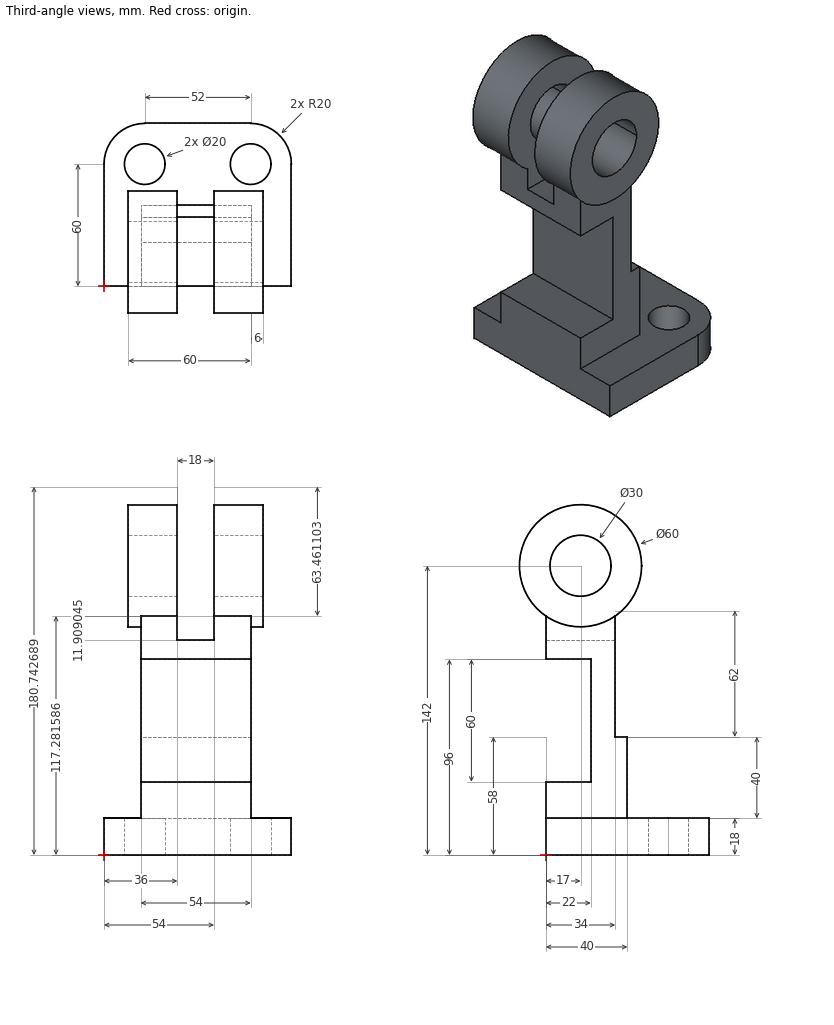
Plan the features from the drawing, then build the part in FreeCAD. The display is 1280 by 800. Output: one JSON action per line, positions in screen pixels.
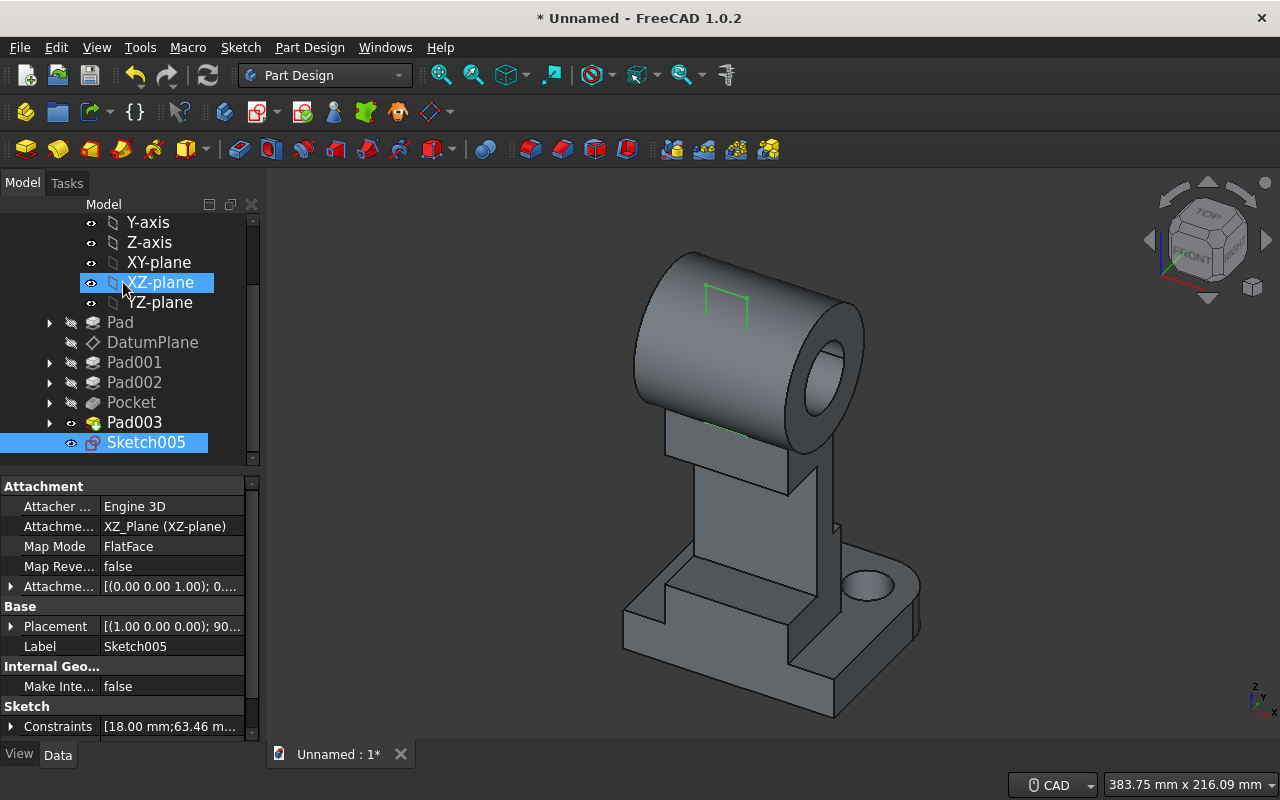
{"action": "left_click", "coordinate": [240, 150]}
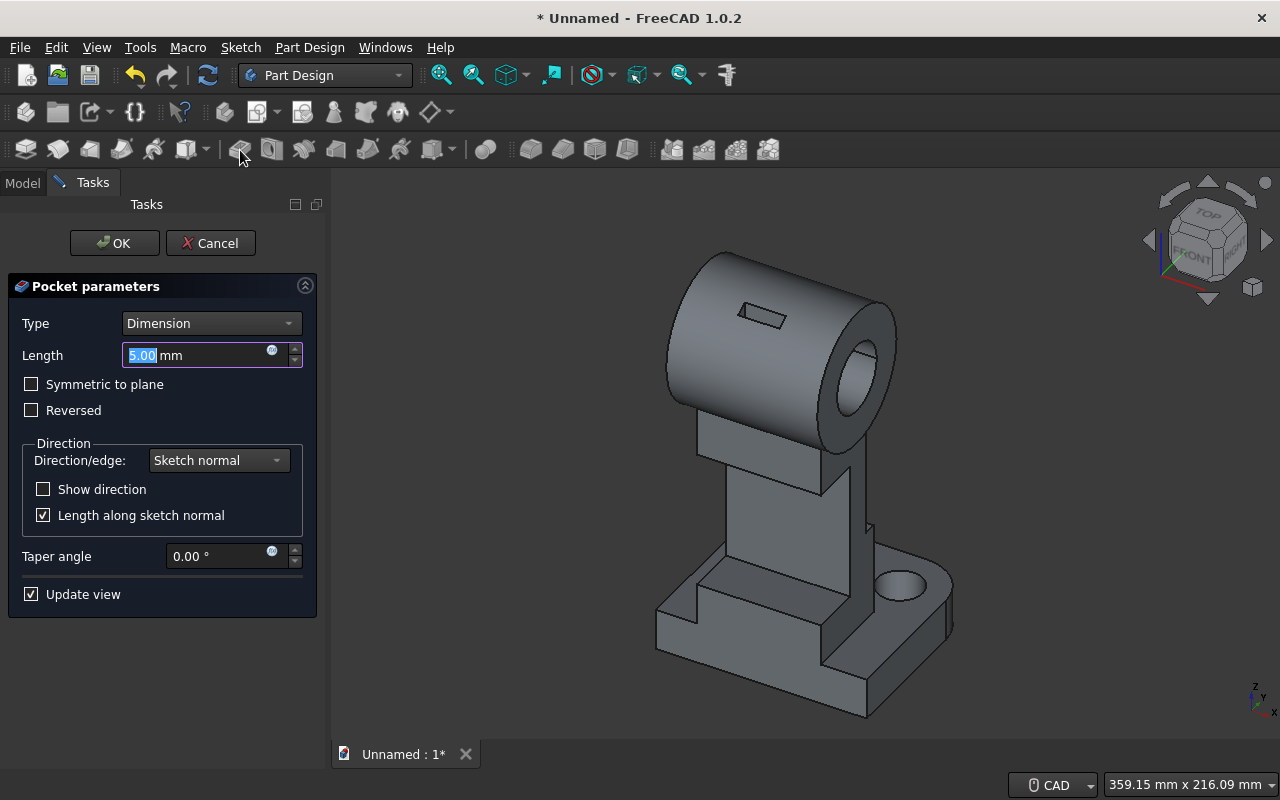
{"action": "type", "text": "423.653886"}
{"action": "key", "text": "Tab"}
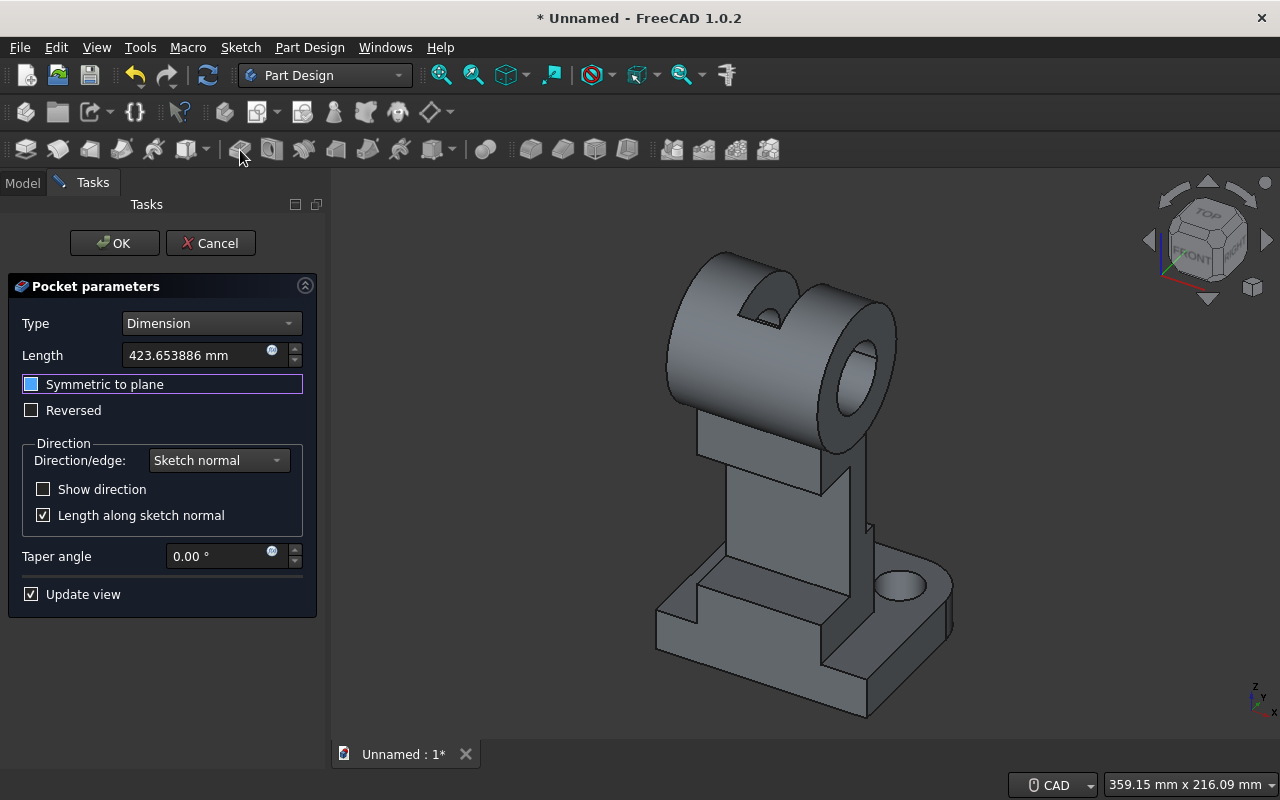
{"action": "left_click", "coordinate": [30, 384]}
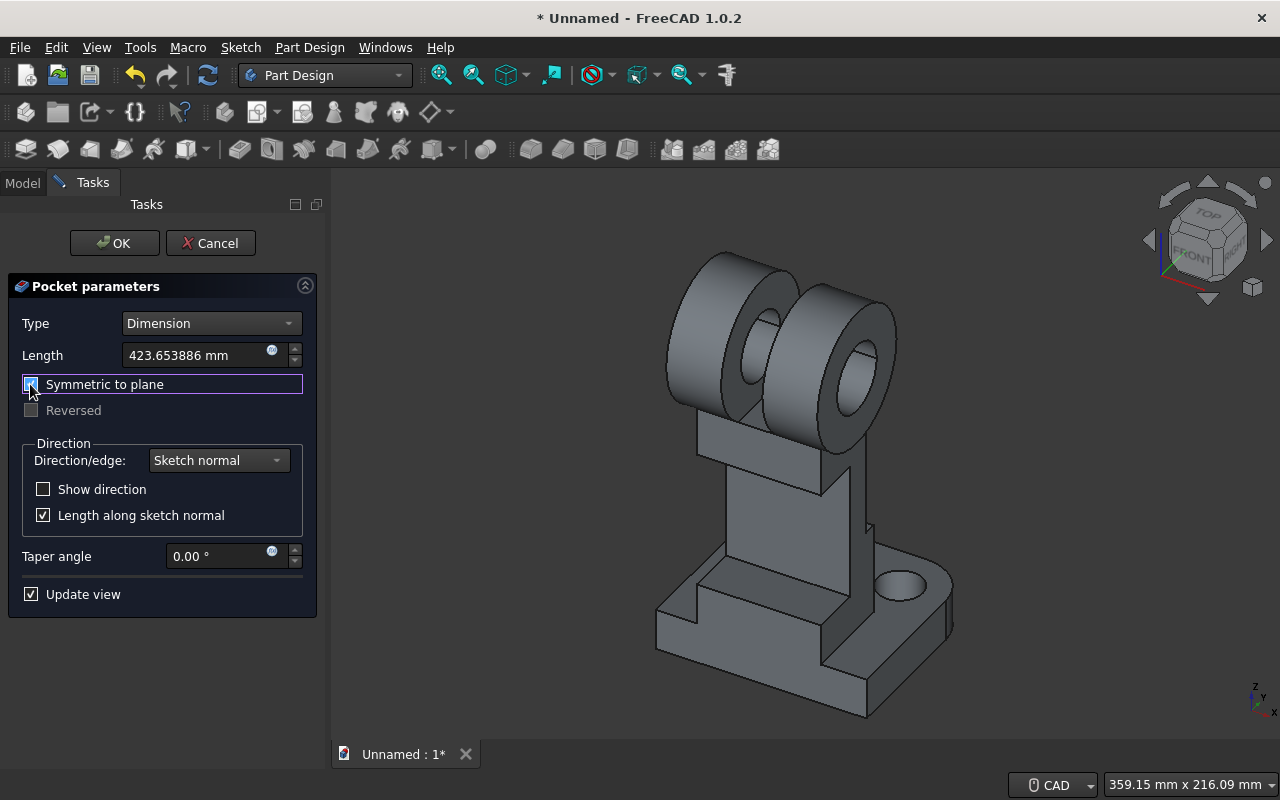
{"action": "left_click", "coordinate": [115, 243]}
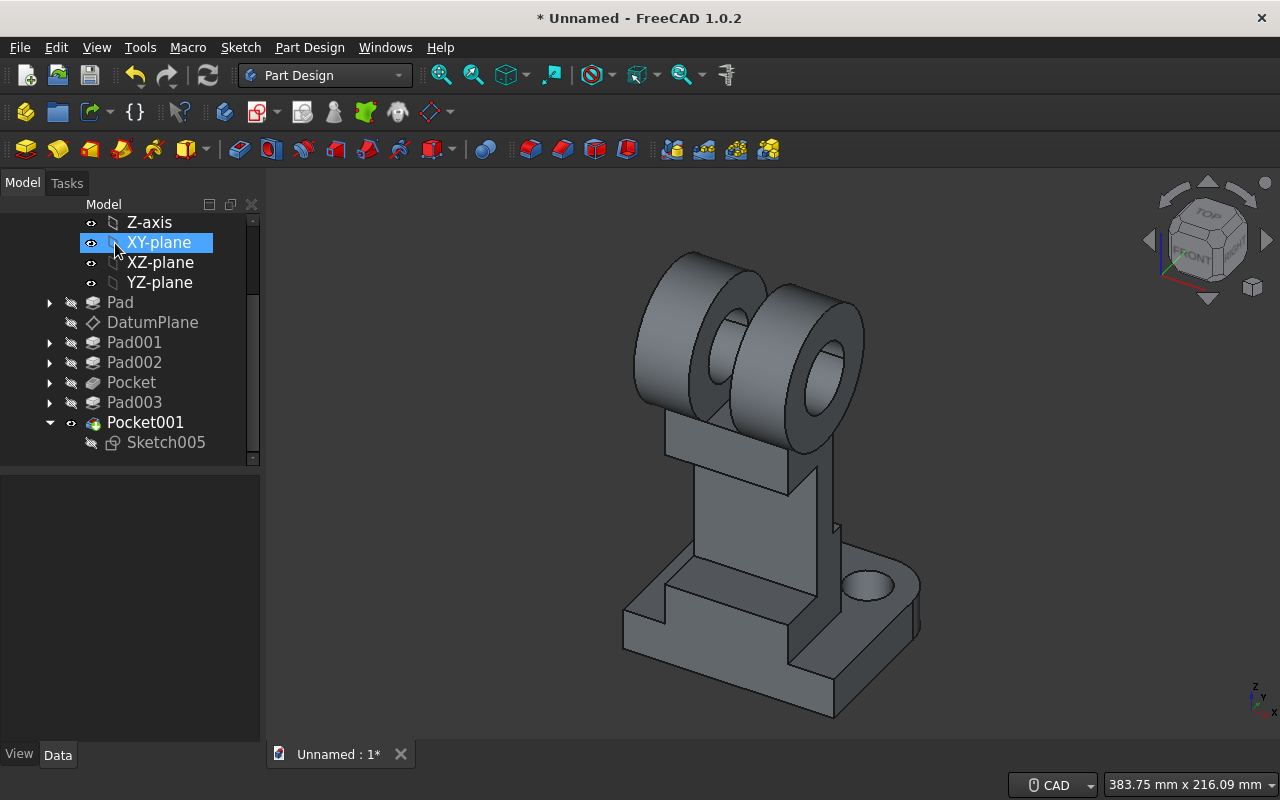
{"action": "key", "text": "4"}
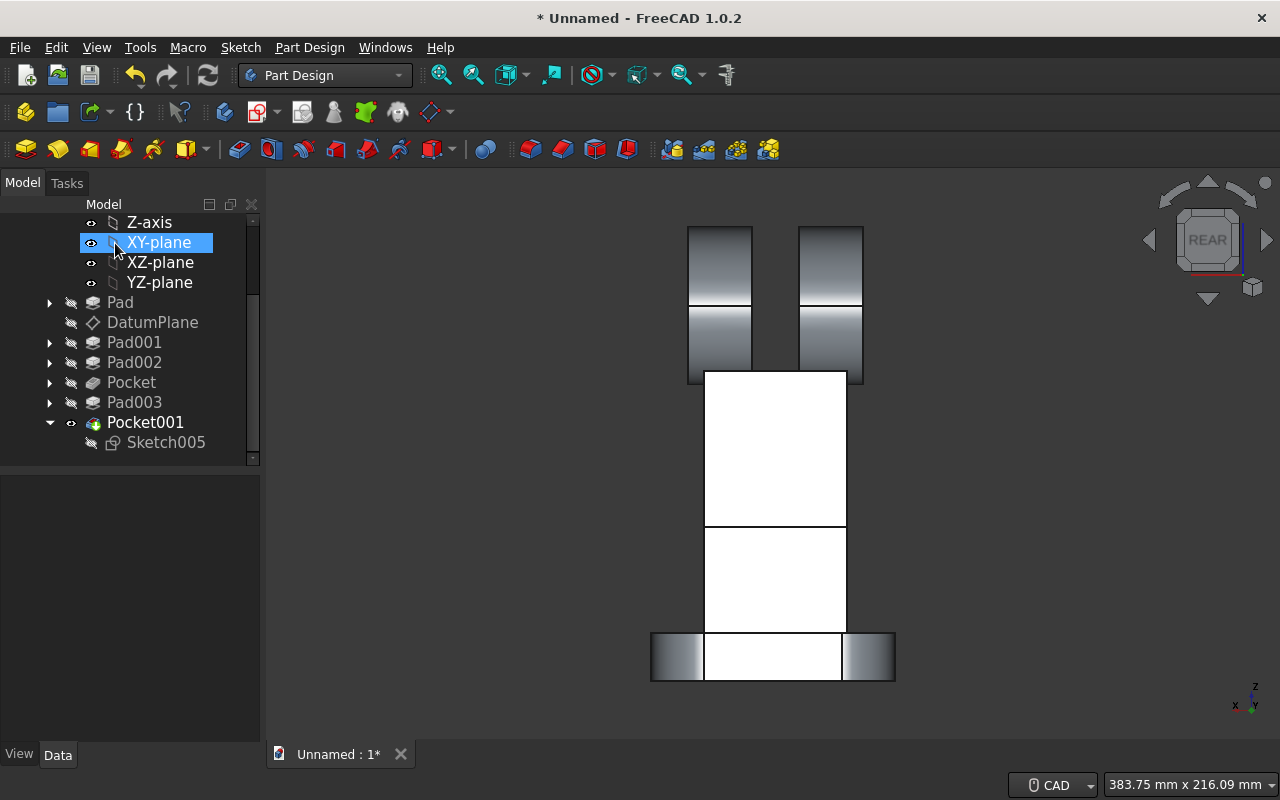
{"action": "left_click", "coordinate": [776, 448]}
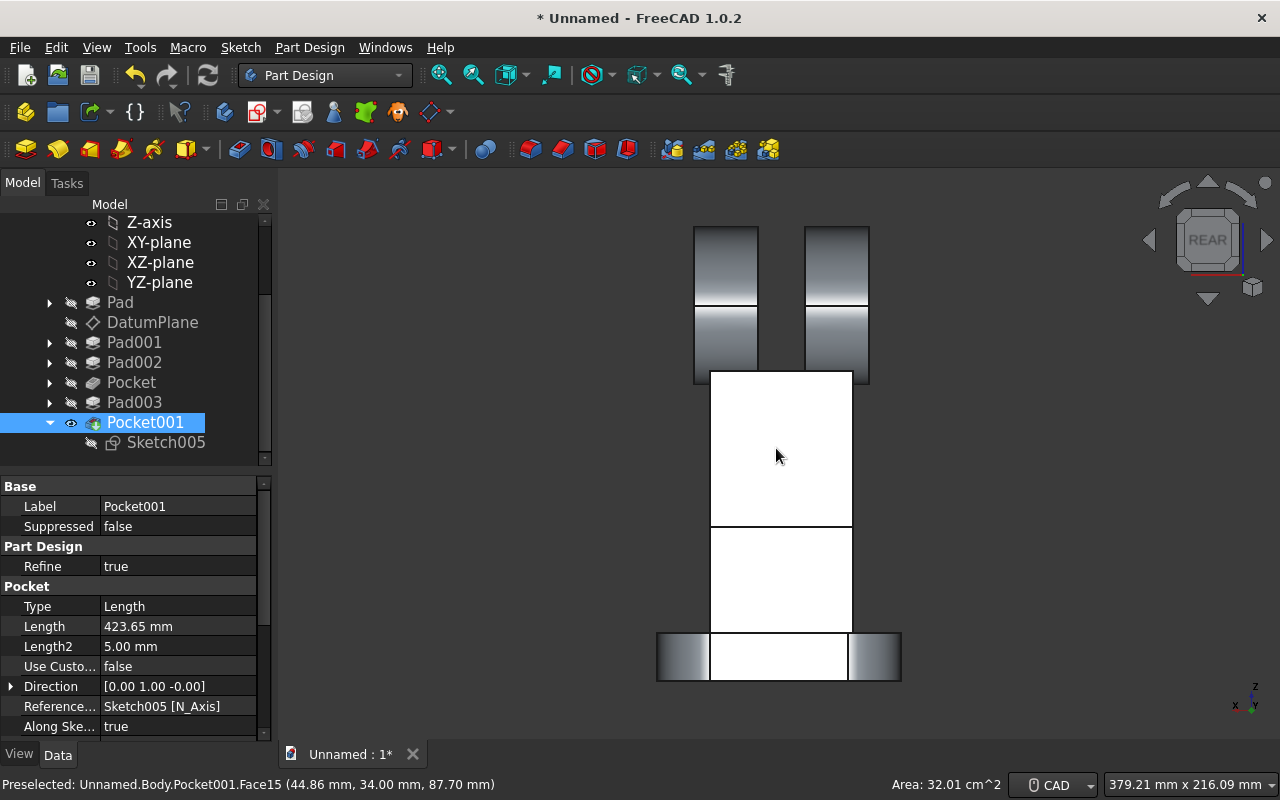
{"action": "left_click", "coordinate": [258, 112]}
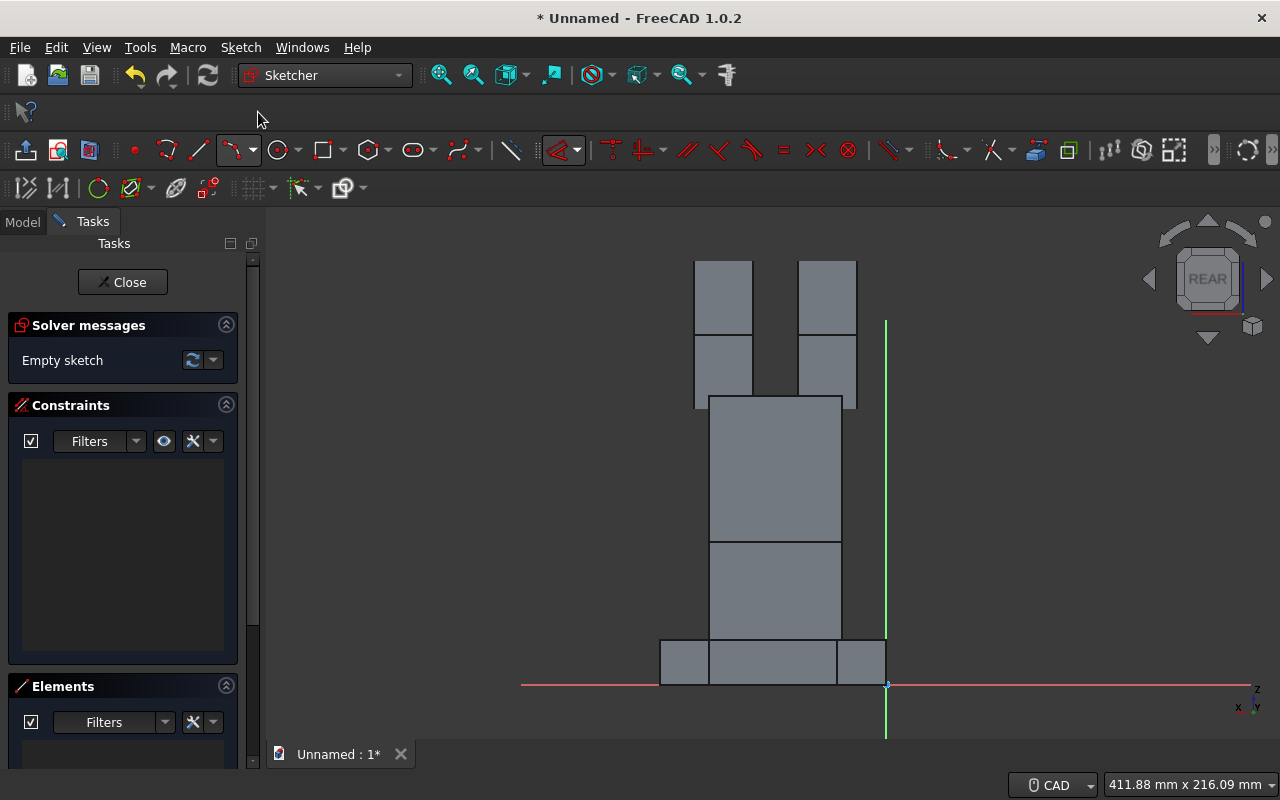
{"action": "scroll", "coordinate": [783, 404], "scroll_direction": "up", "scroll_amount": 12}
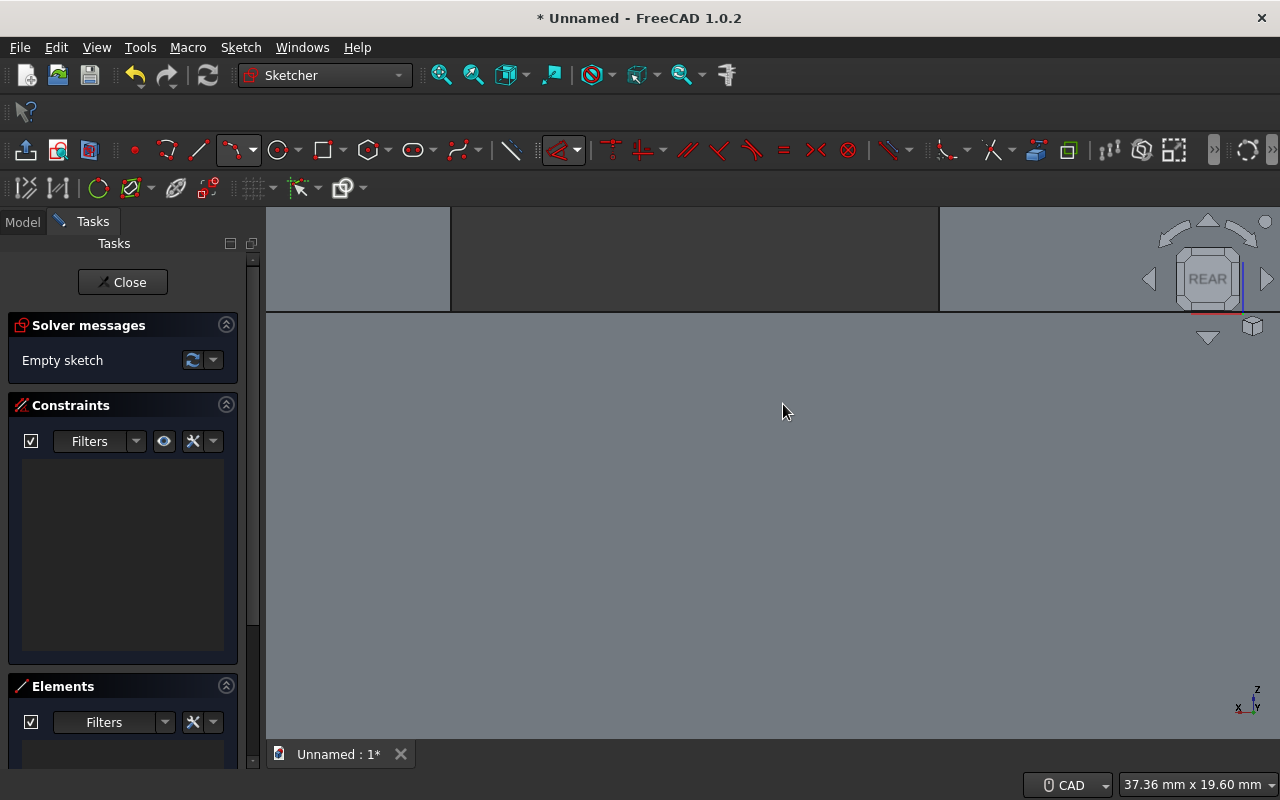
{"action": "left_click", "coordinate": [324, 150]}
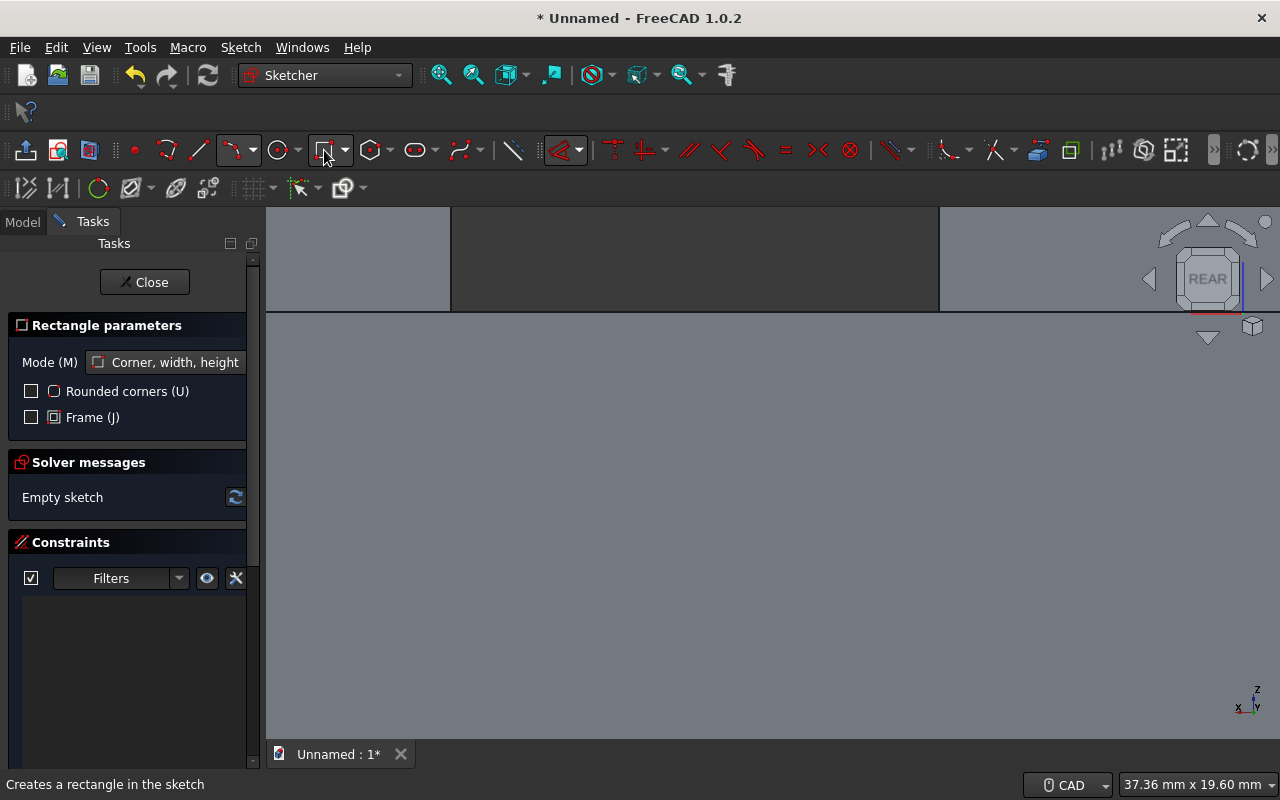
{"action": "left_click", "coordinate": [451, 312]}
{"action": "mouse_move", "coordinate": [939, 635]}